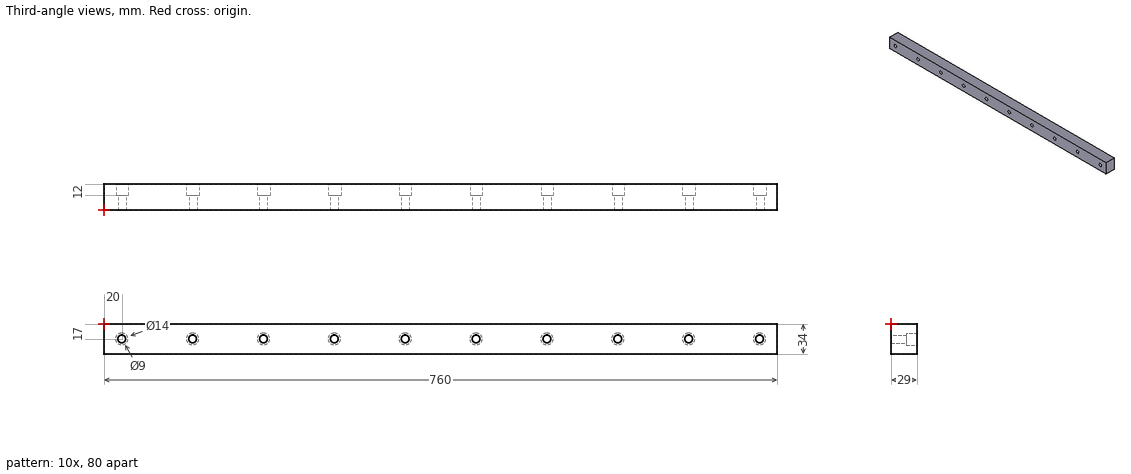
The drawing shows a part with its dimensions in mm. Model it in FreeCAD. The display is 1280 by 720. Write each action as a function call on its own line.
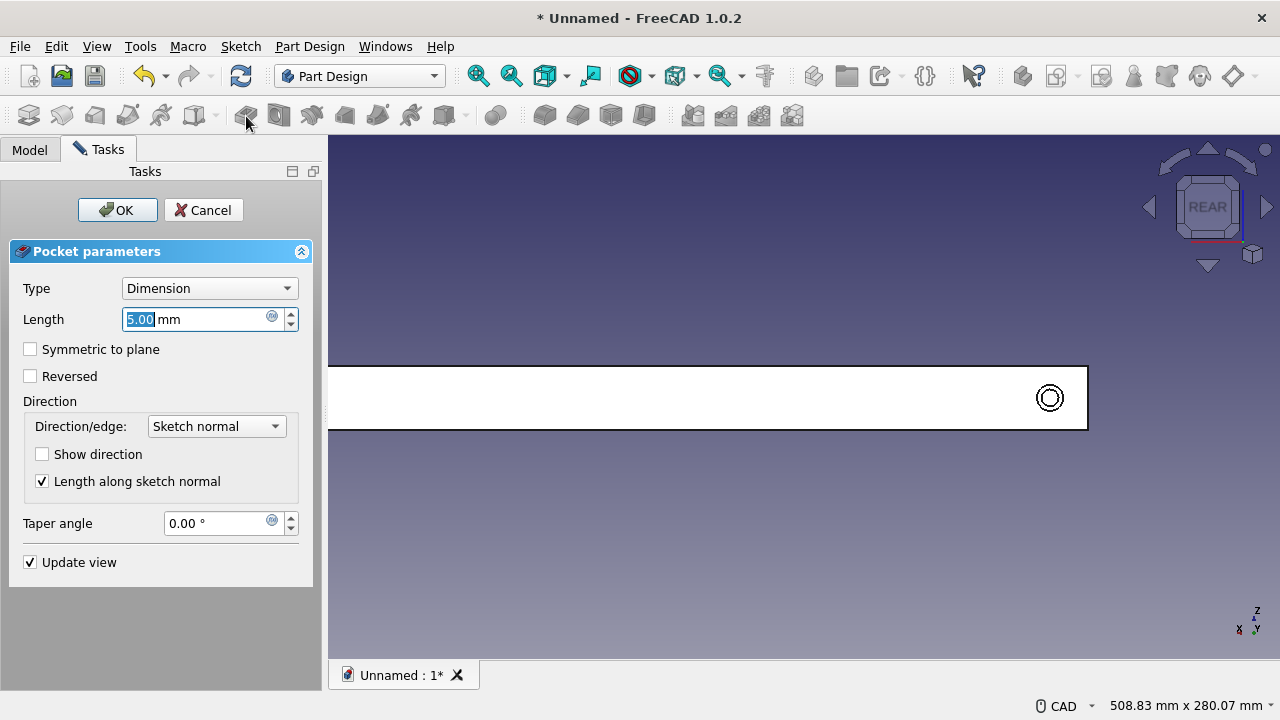
click(210, 288)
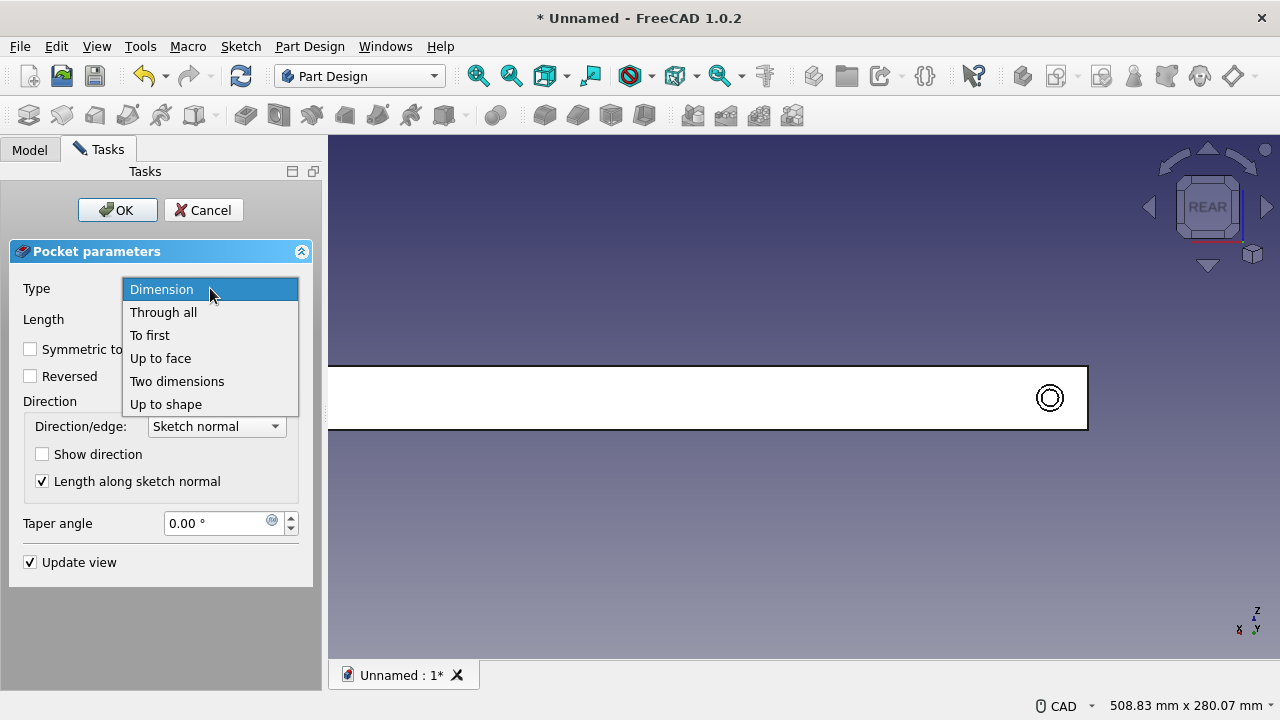
click(208, 312)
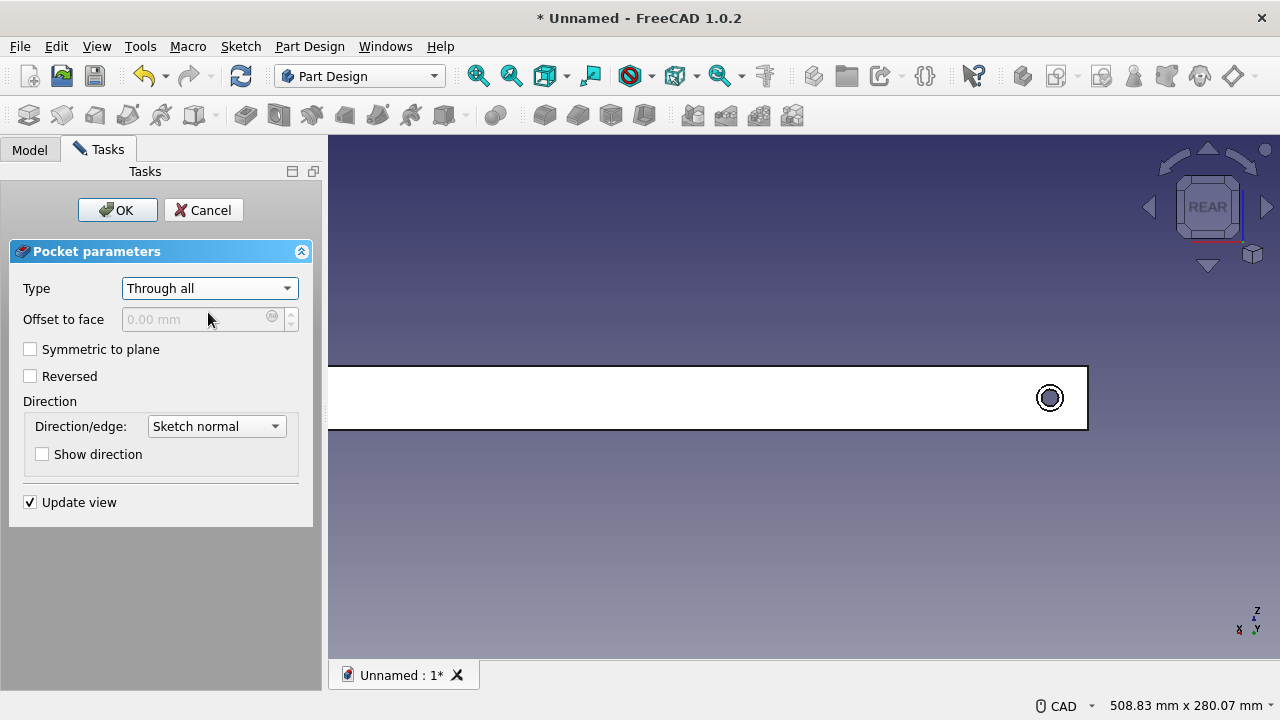
click(118, 210)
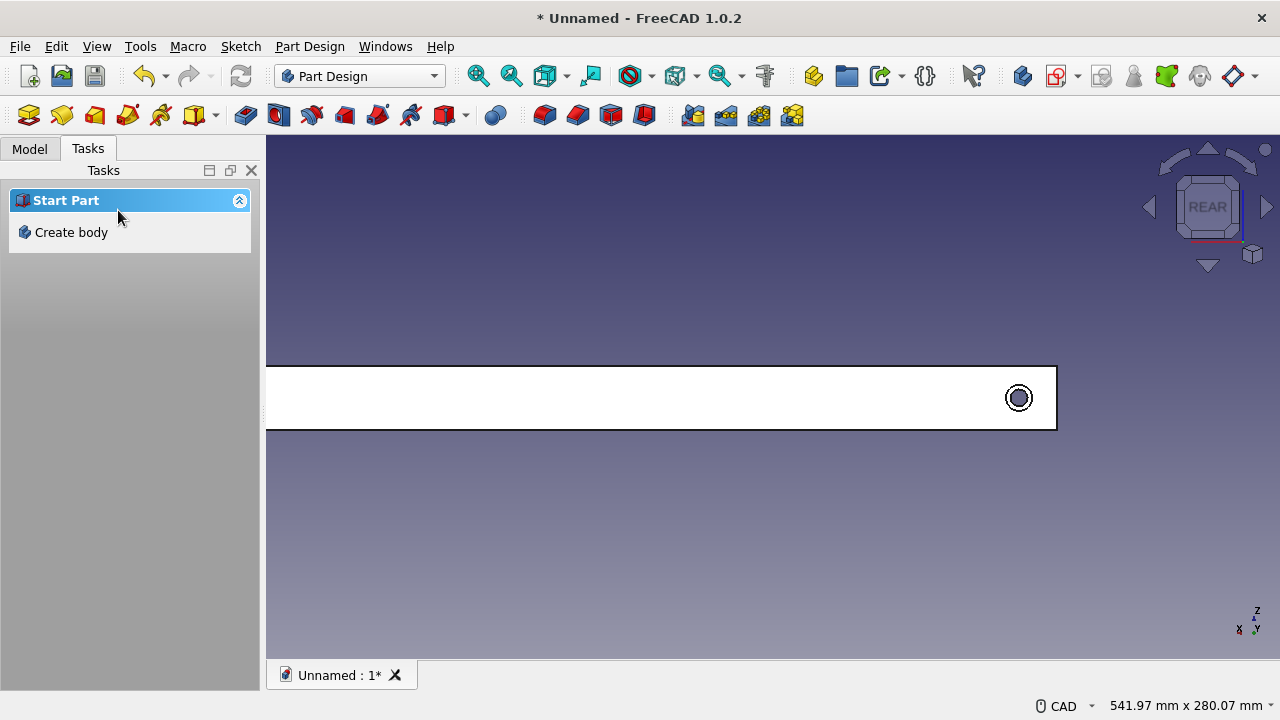
key(v)
key(f)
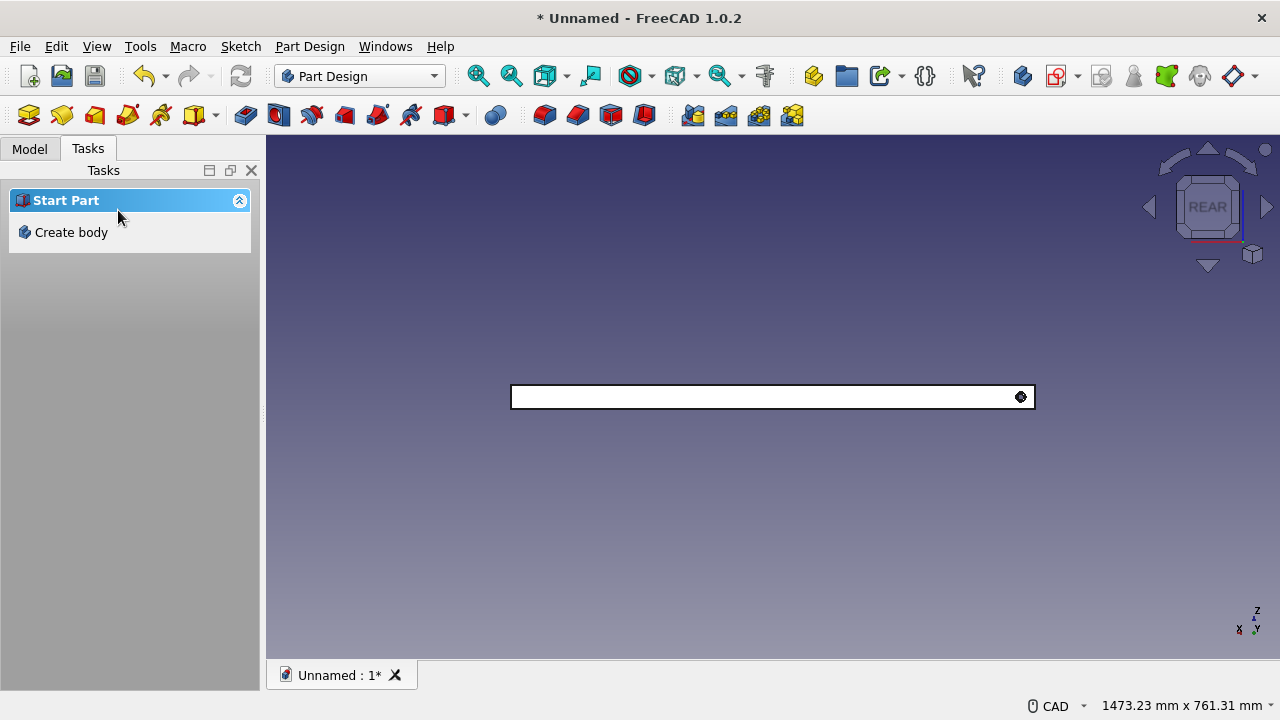
click(30, 148)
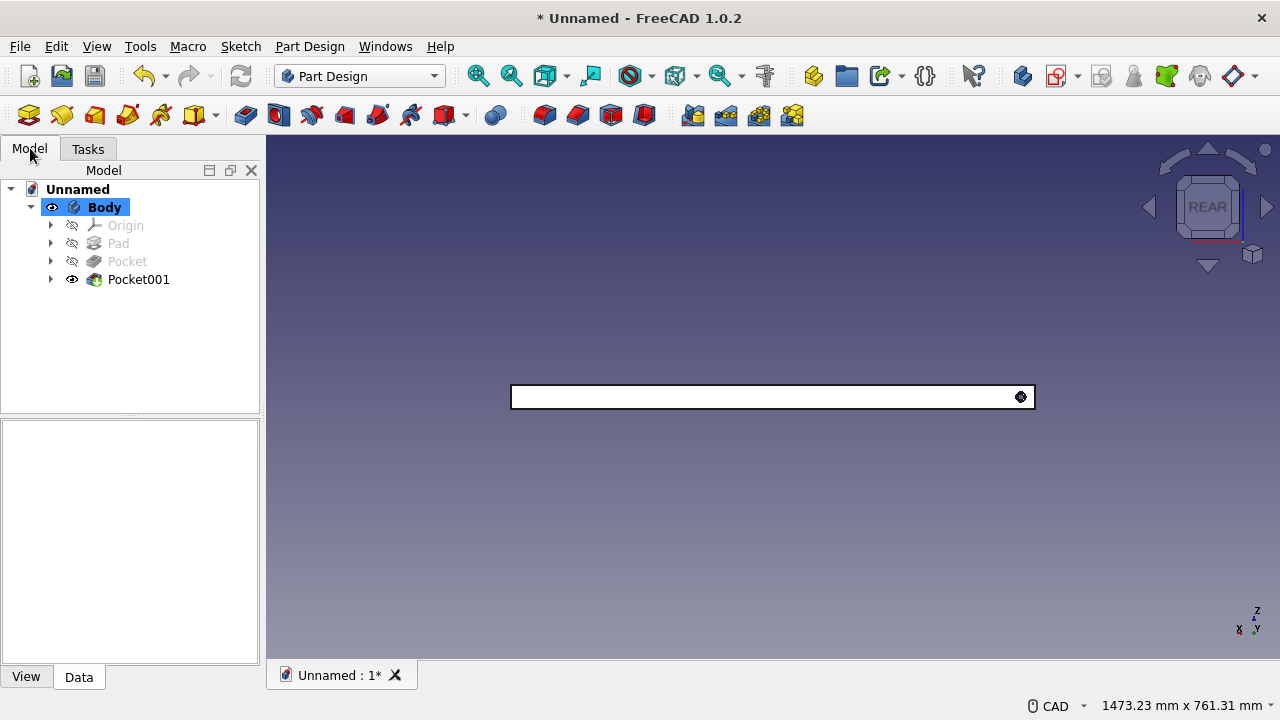
click(117, 261)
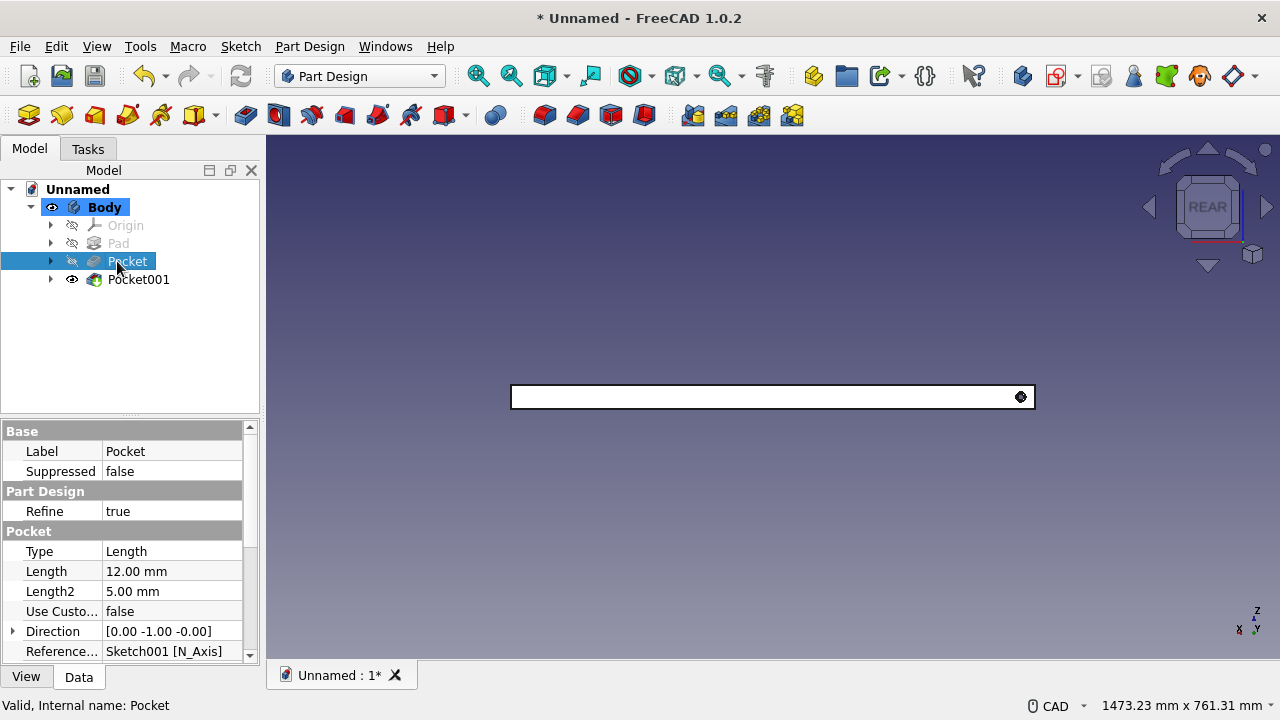
click(117, 279, ctrl)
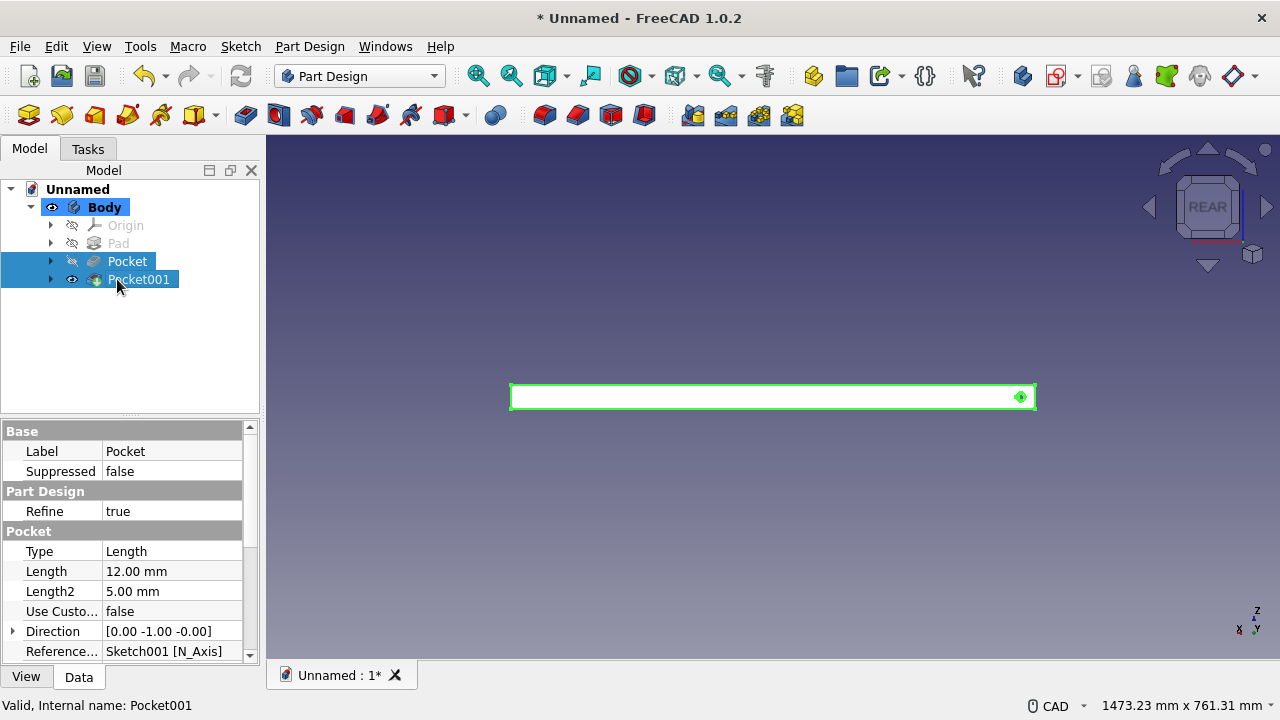
click(726, 116)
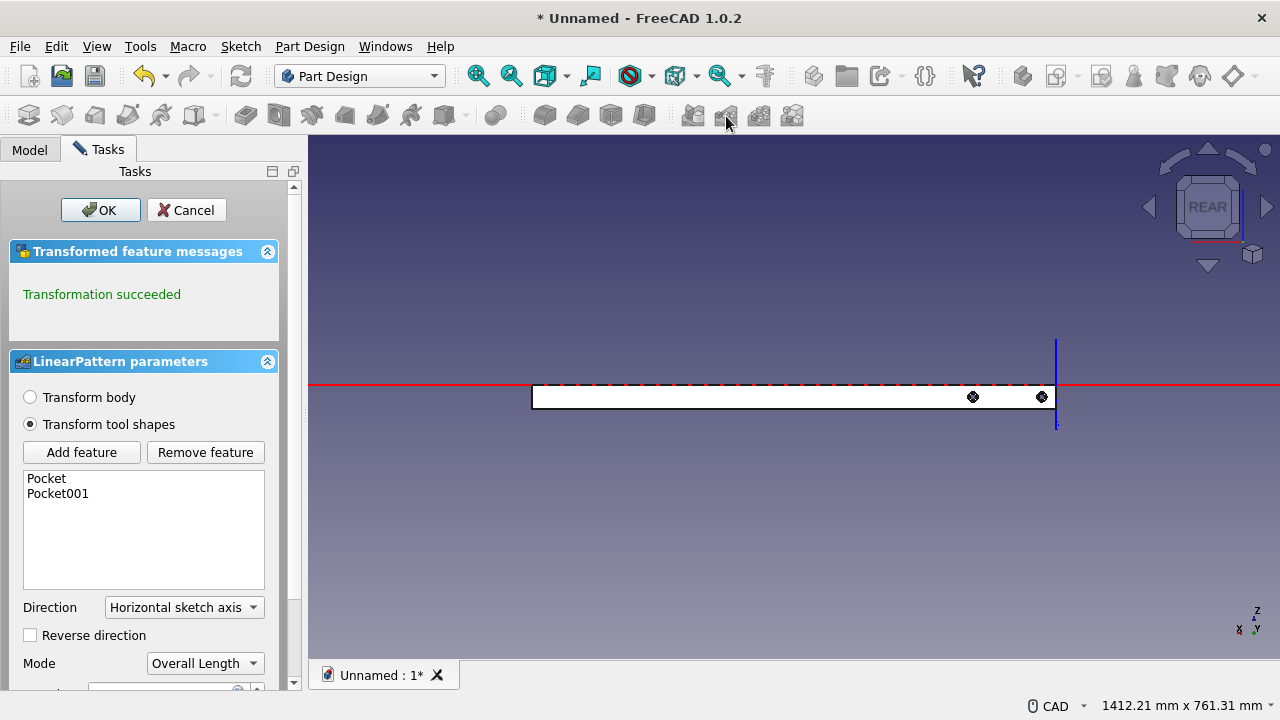
click(185, 608)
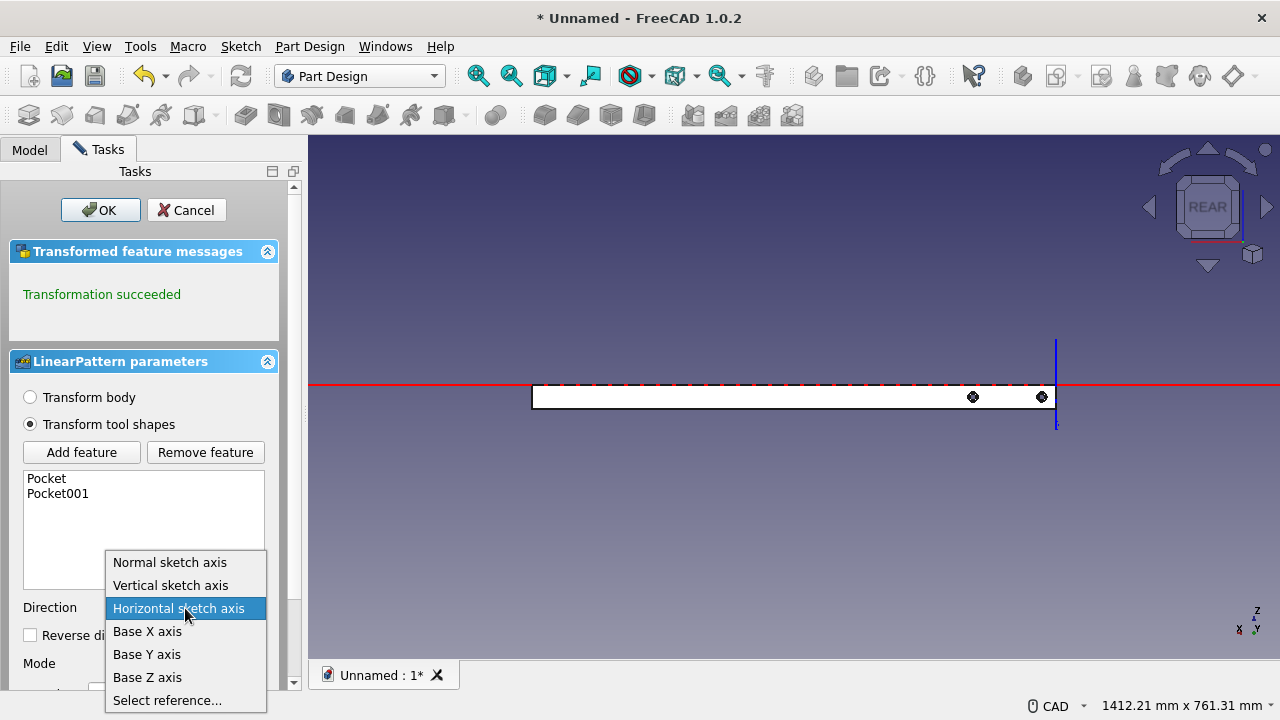
click(184, 632)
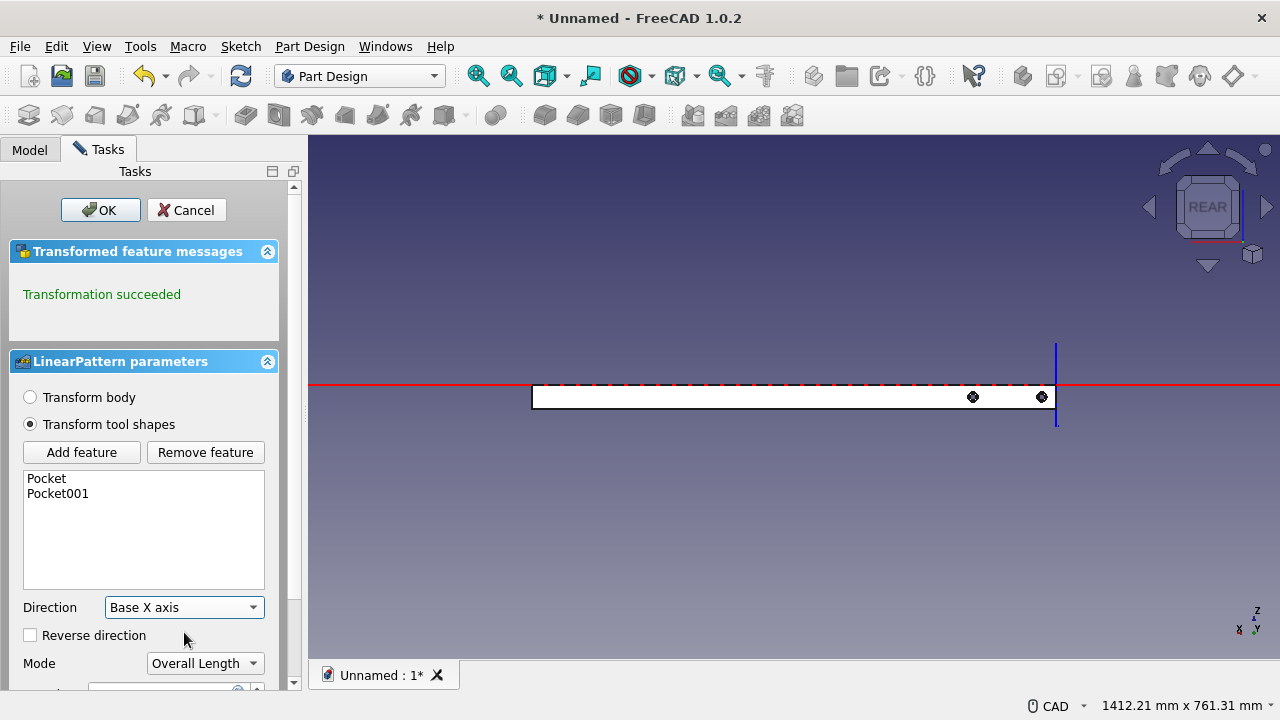
click(206, 664)